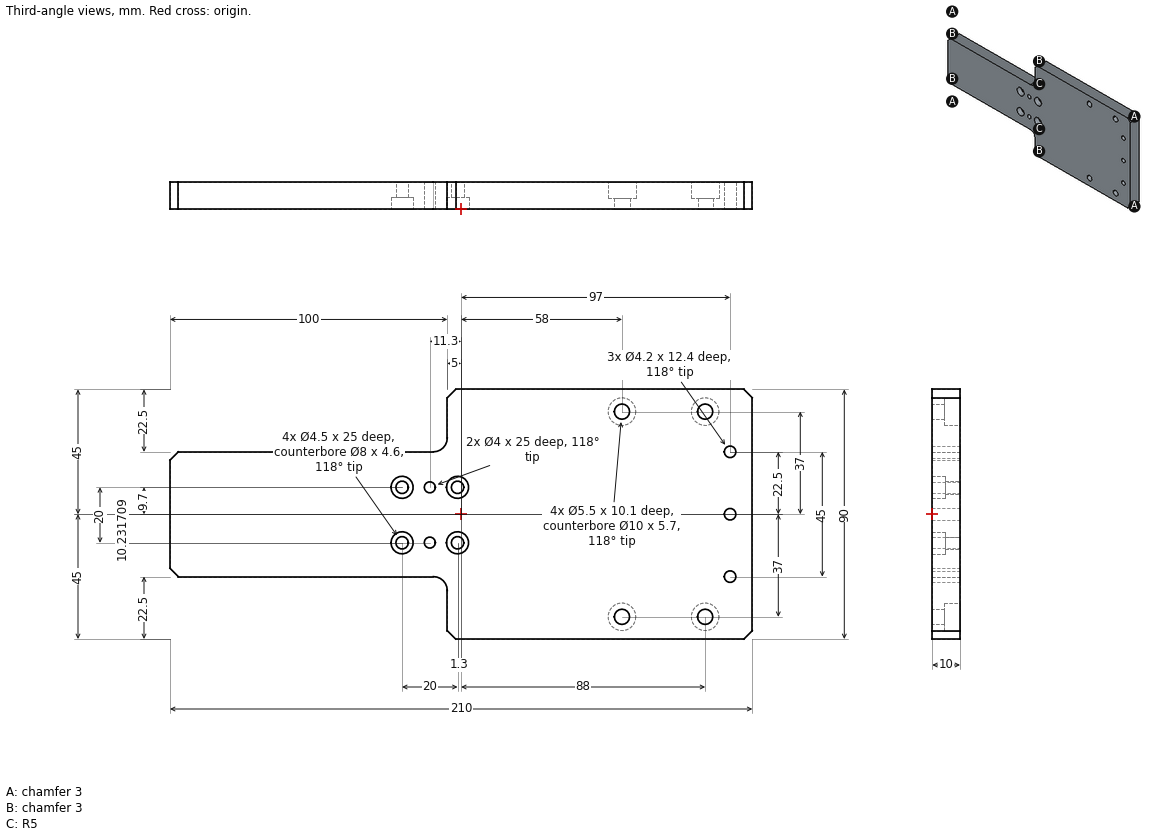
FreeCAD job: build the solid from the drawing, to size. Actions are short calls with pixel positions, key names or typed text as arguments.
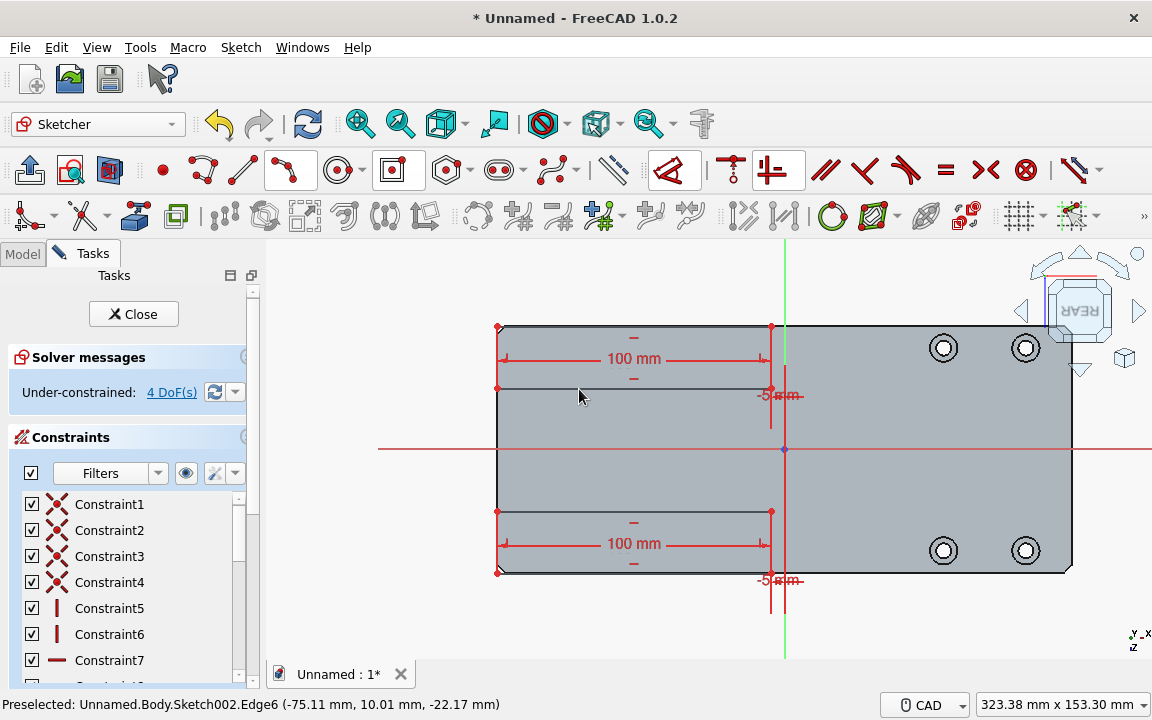
click(497, 574)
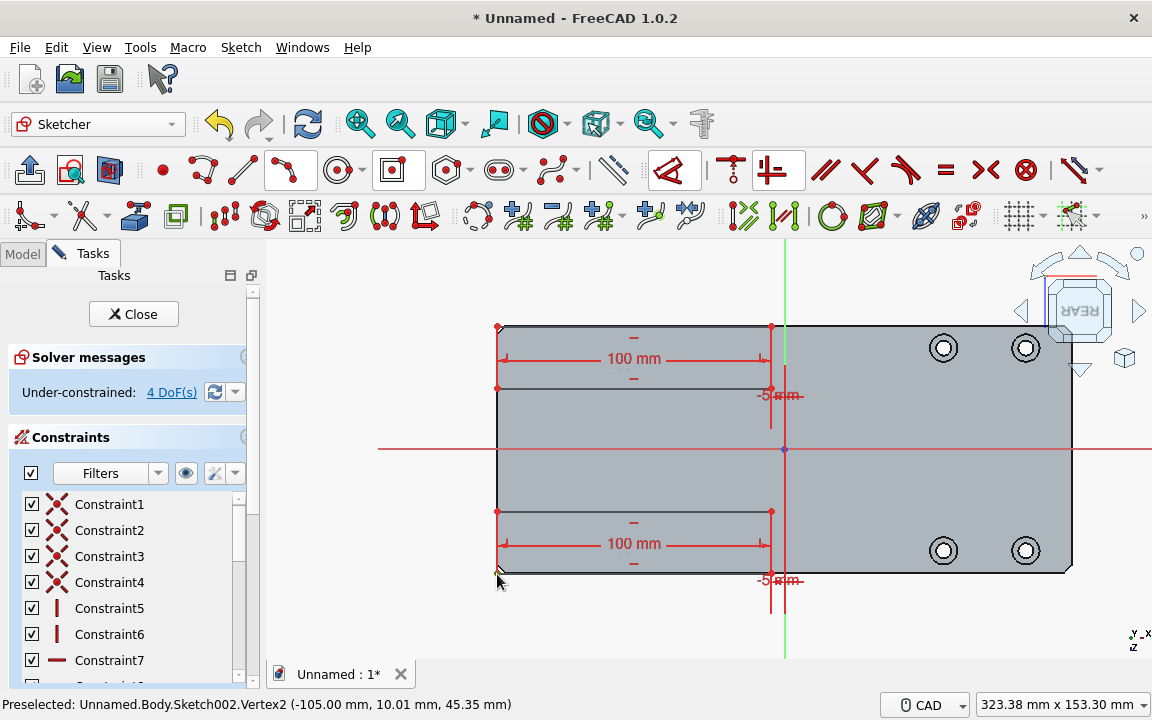
click(696, 170)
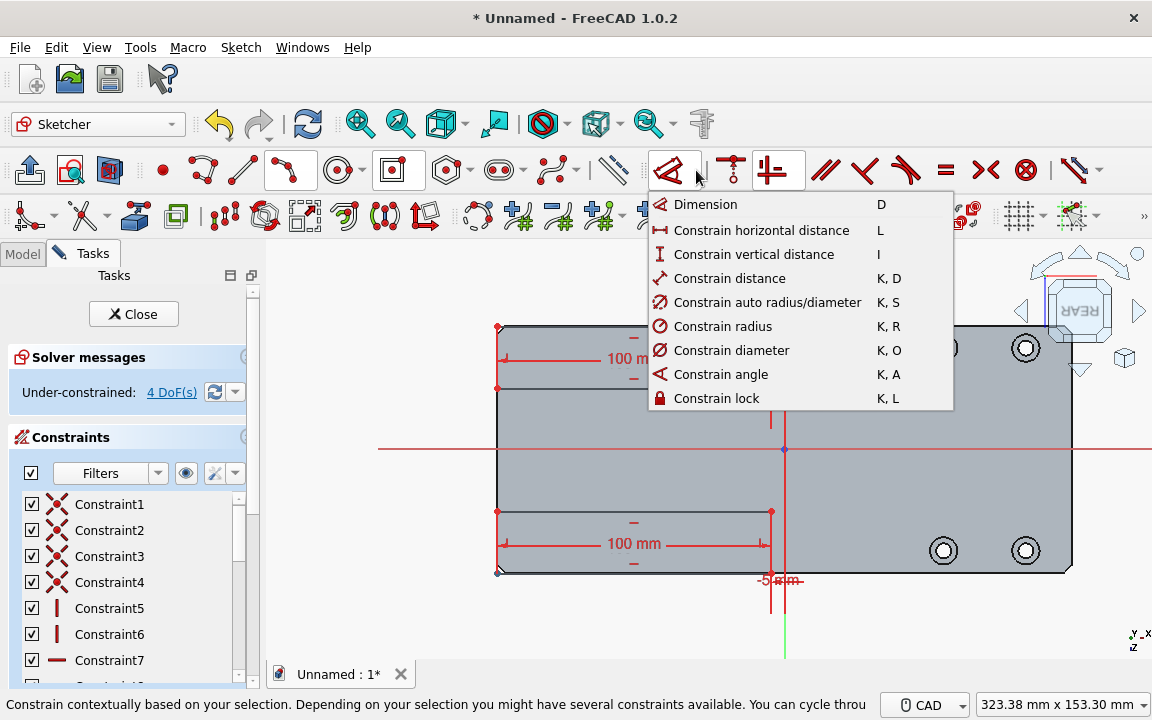
click(801, 254)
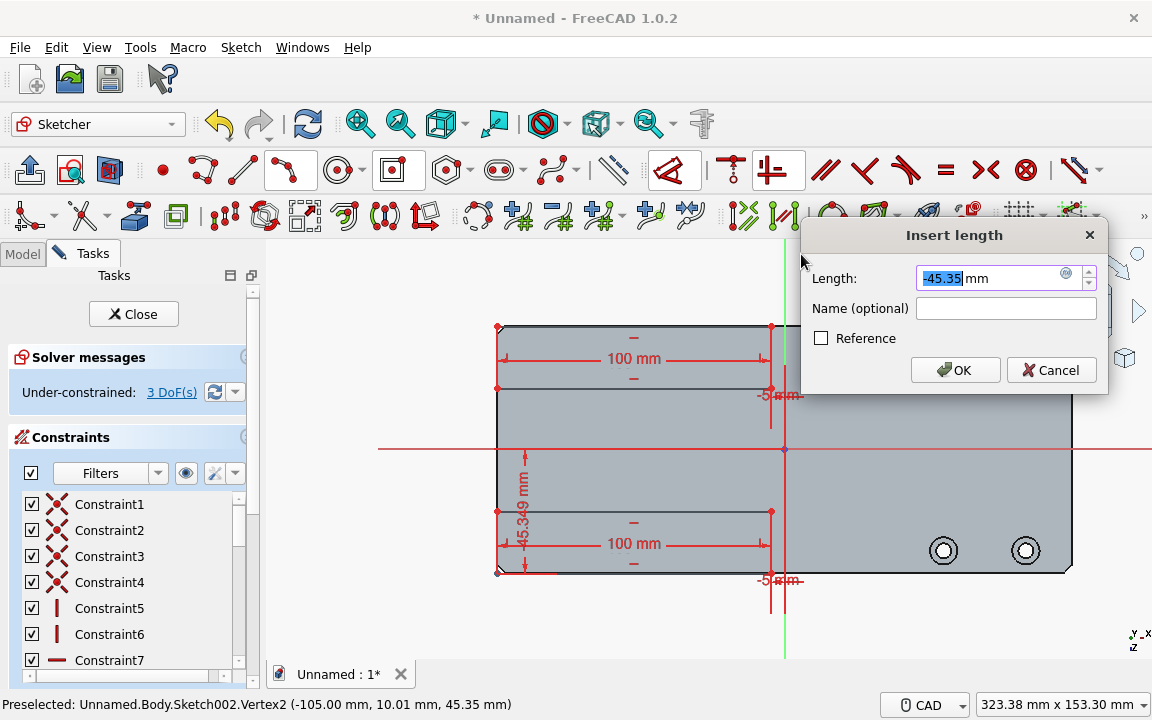
text(-45)
key(Return)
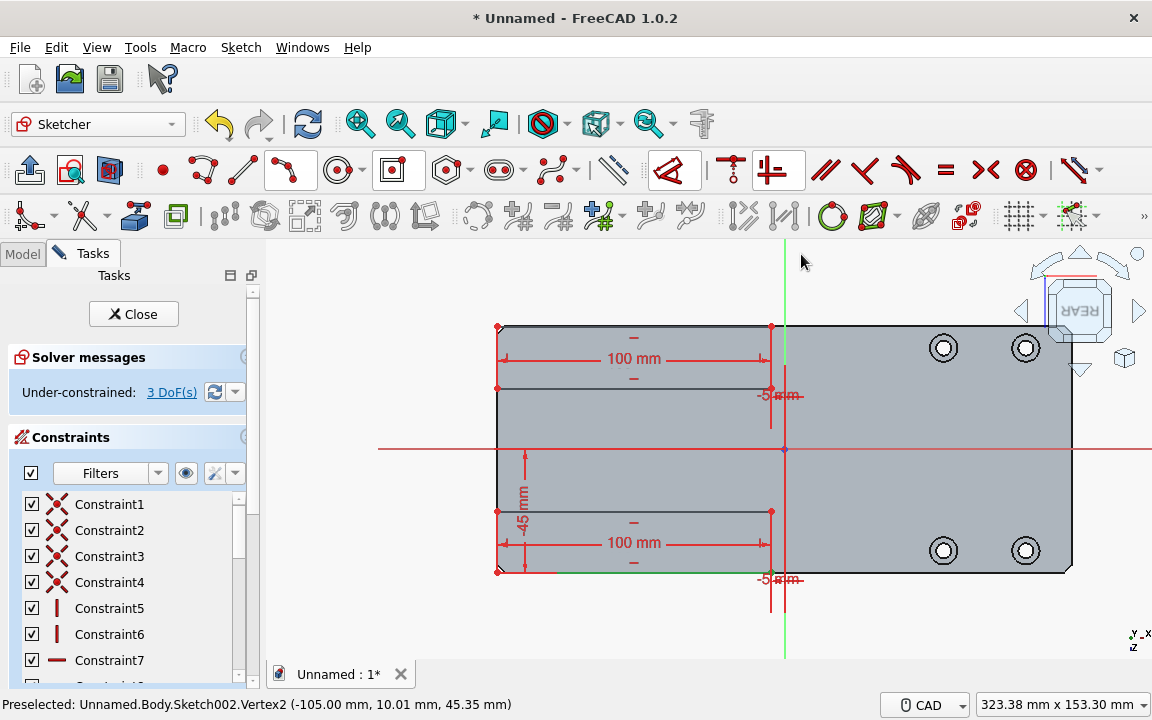
click(497, 327)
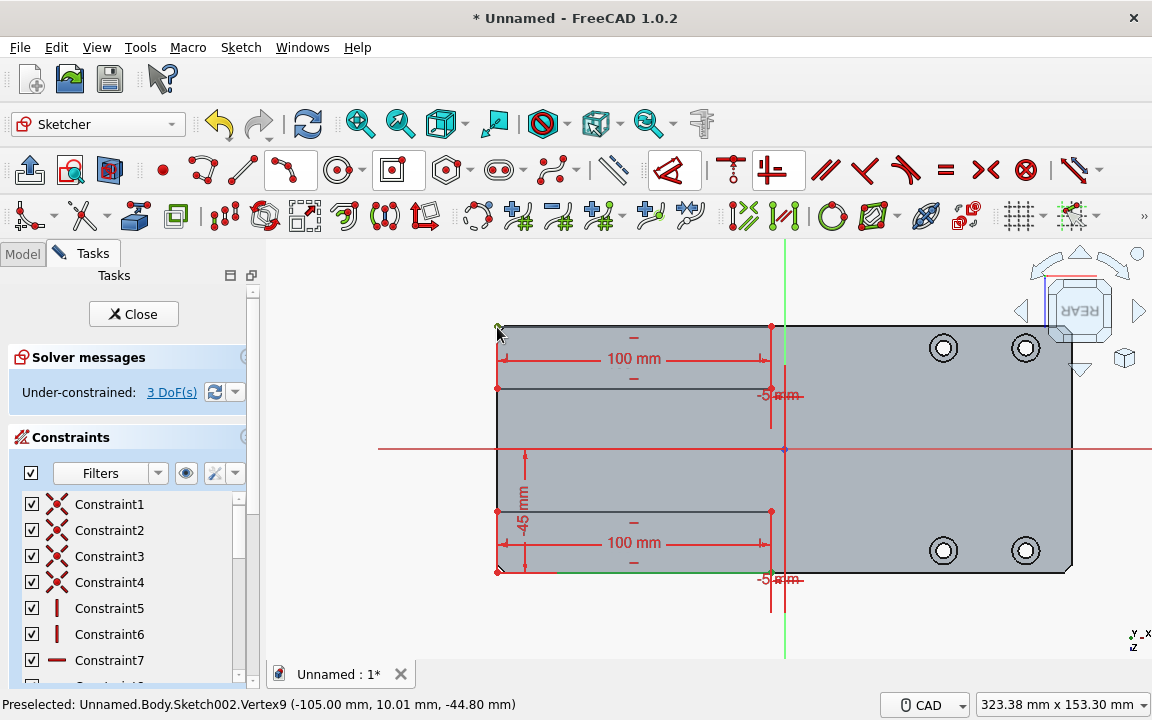
click(696, 170)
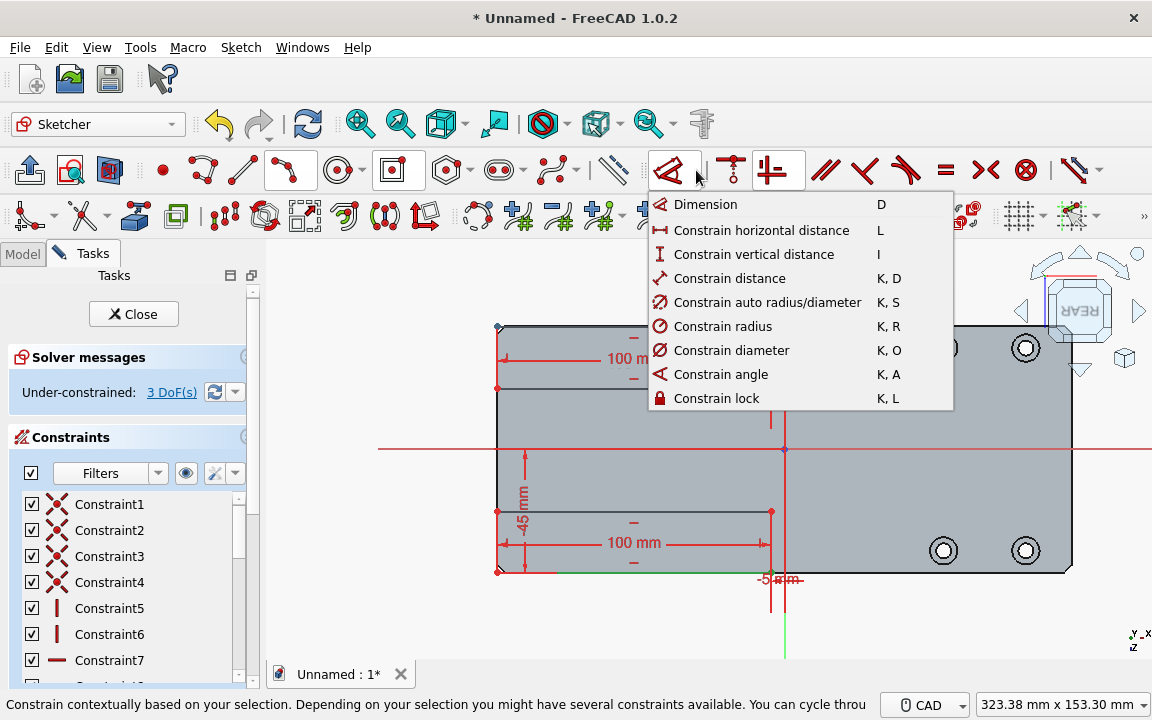
click(801, 254)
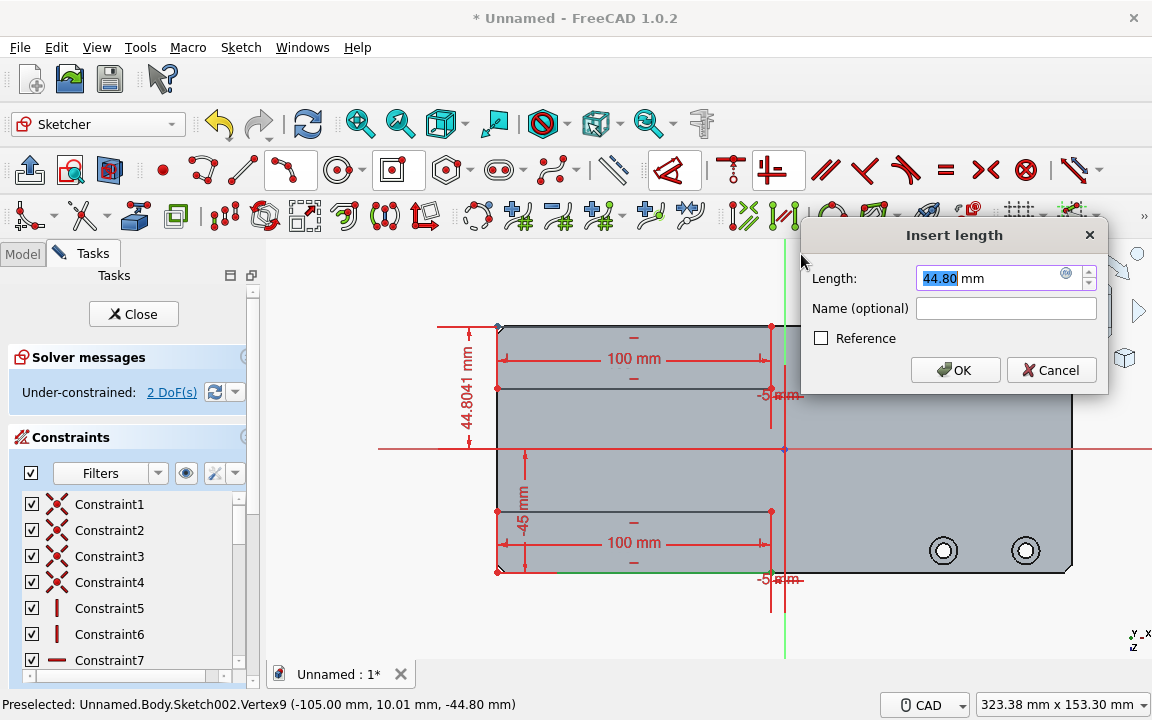
text(45)
key(Return)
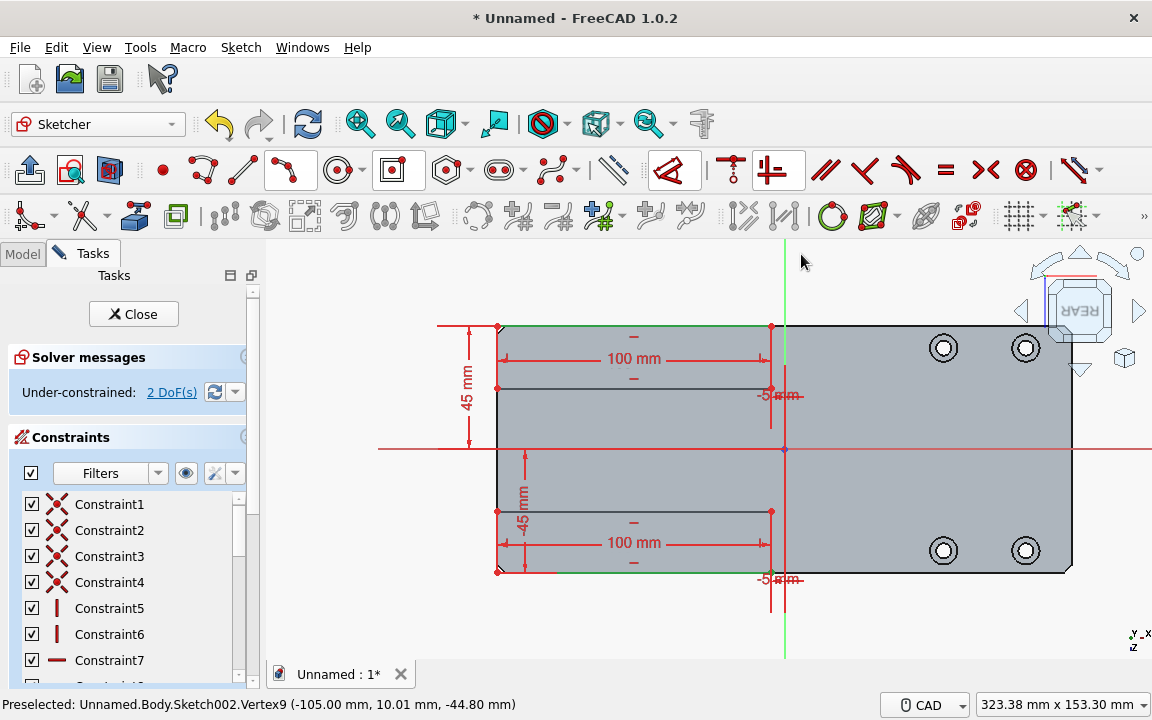
click(497, 530)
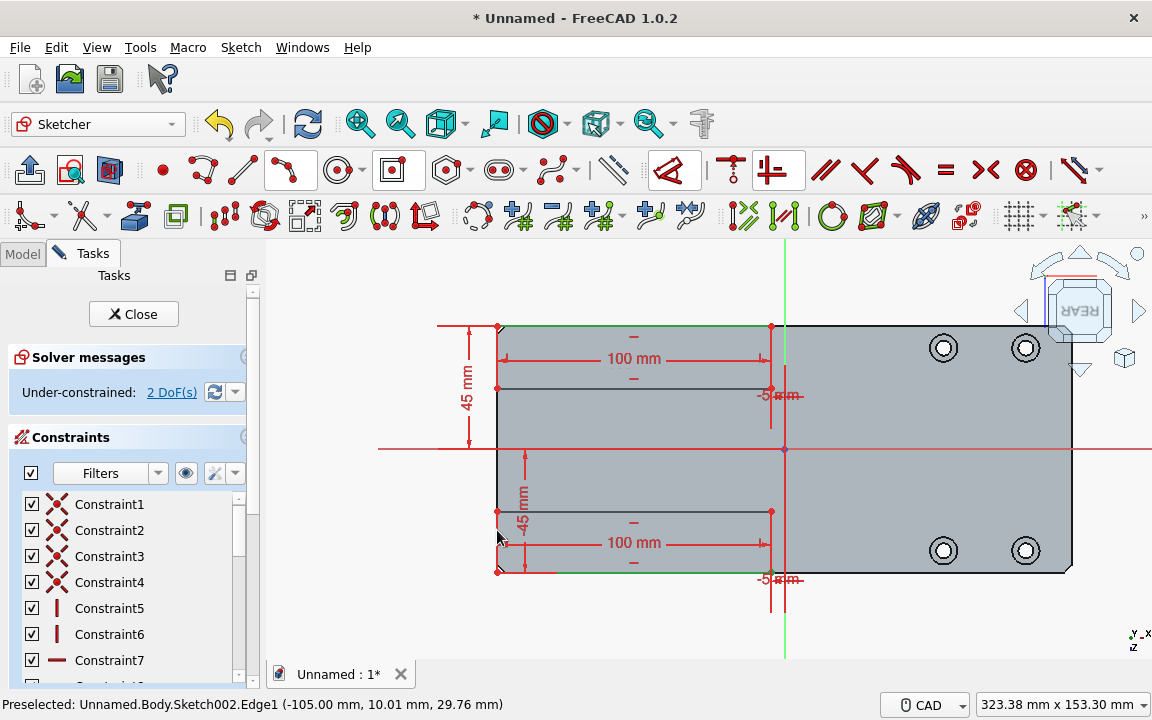
click(696, 170)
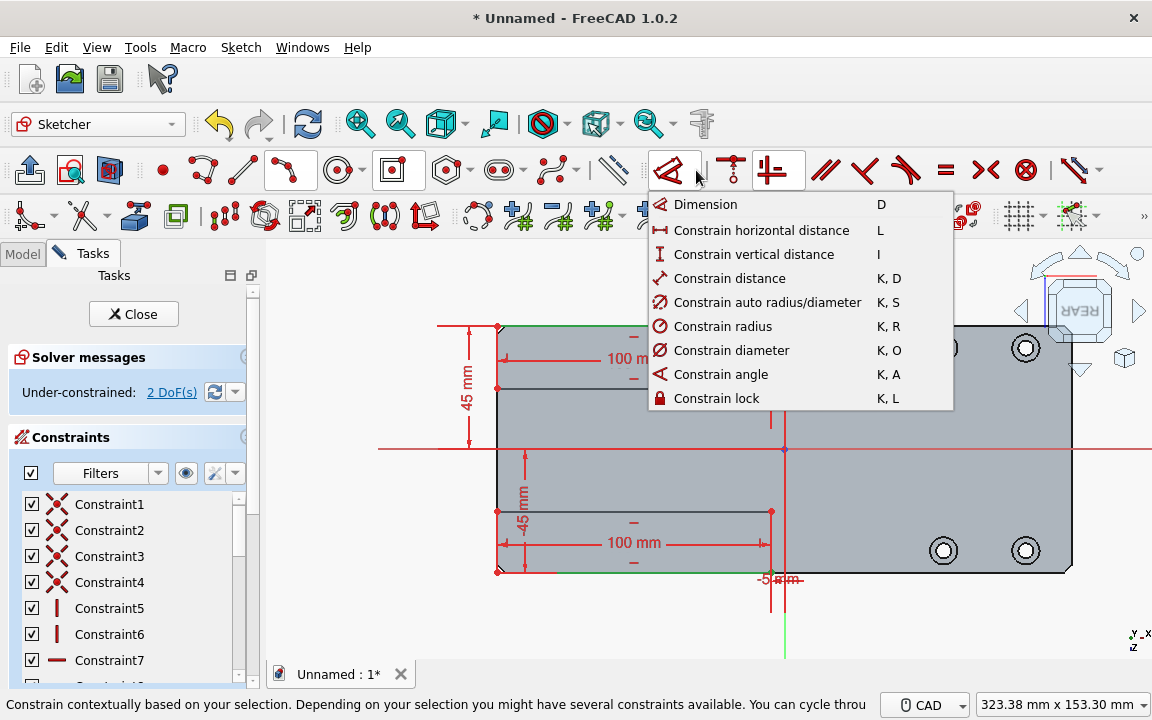
click(801, 254)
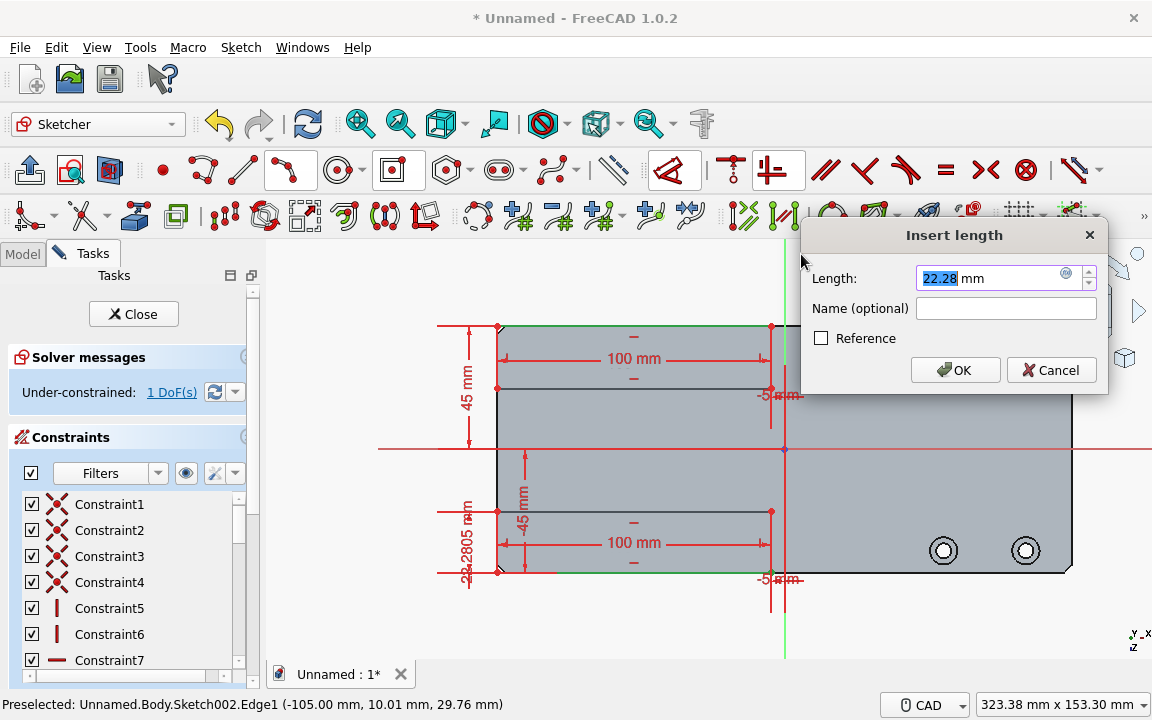
text(22.5)
key(Return)